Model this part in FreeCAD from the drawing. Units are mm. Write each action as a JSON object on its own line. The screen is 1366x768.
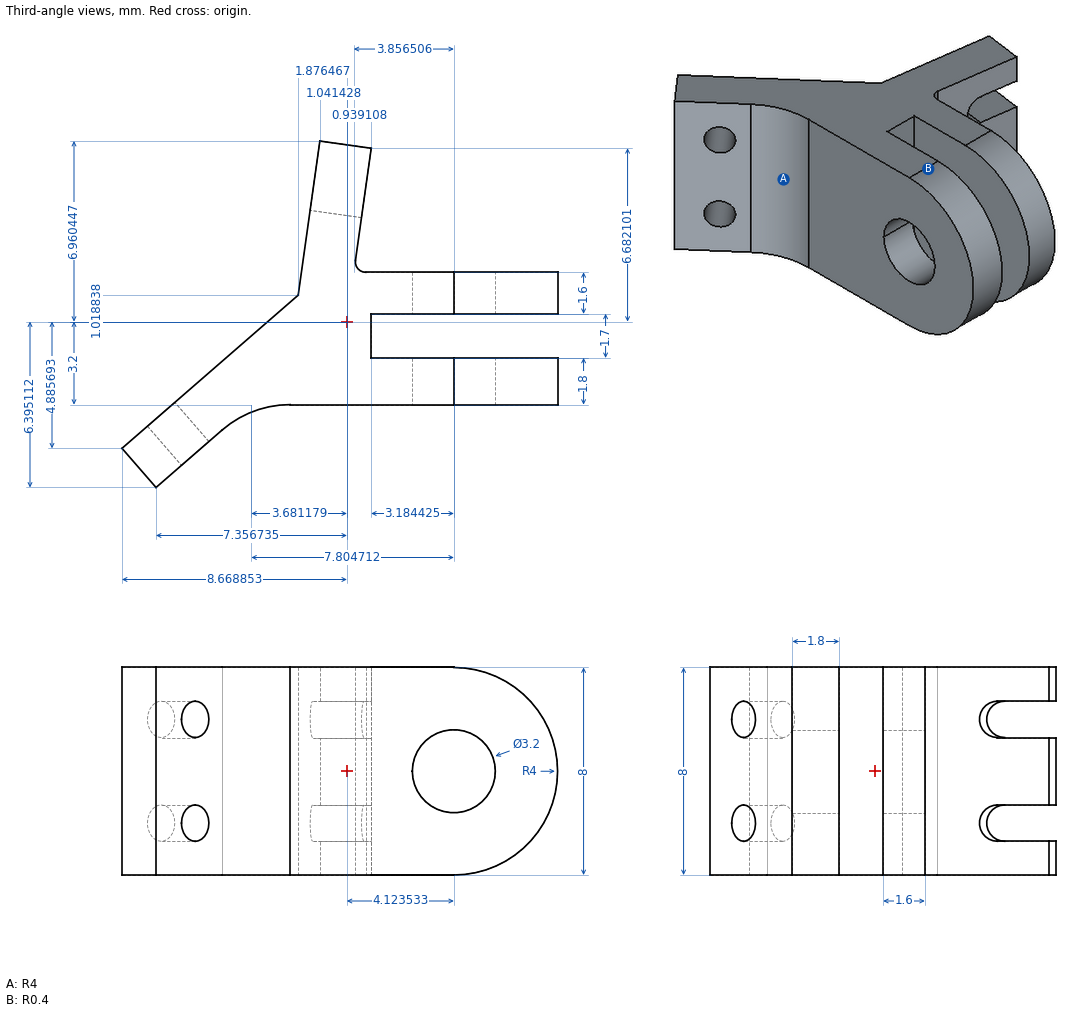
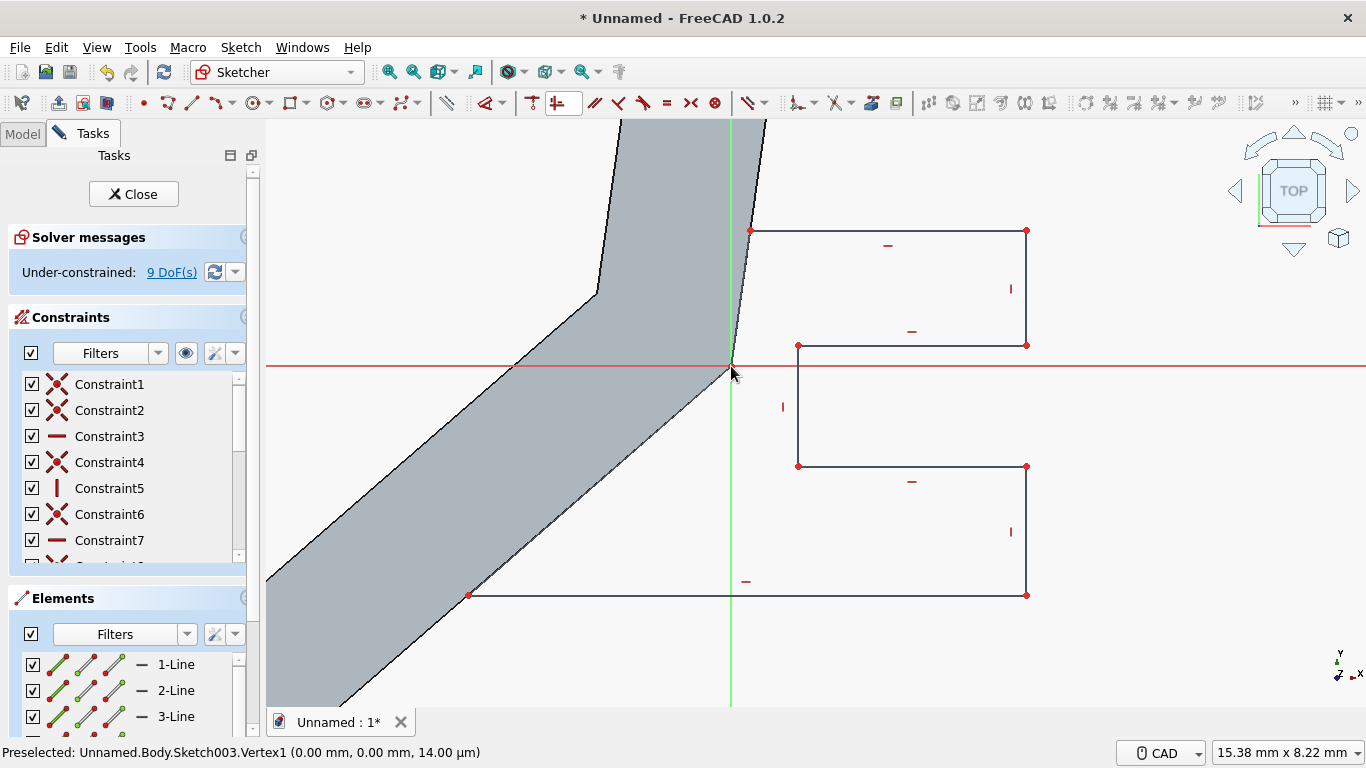
{"action": "left_click", "coordinate": [486, 104]}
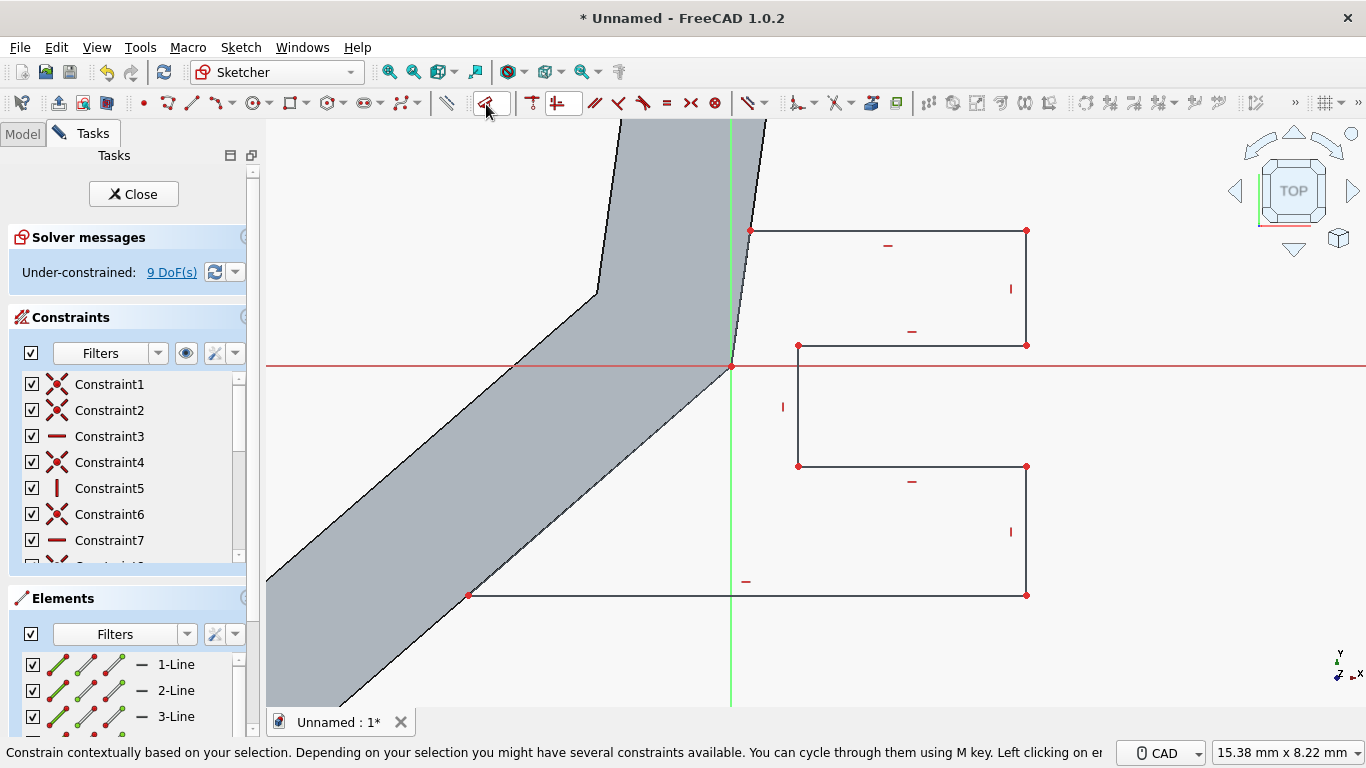
{"action": "left_click", "coordinate": [1026, 557]}
{"action": "left_click", "coordinate": [1060, 532]}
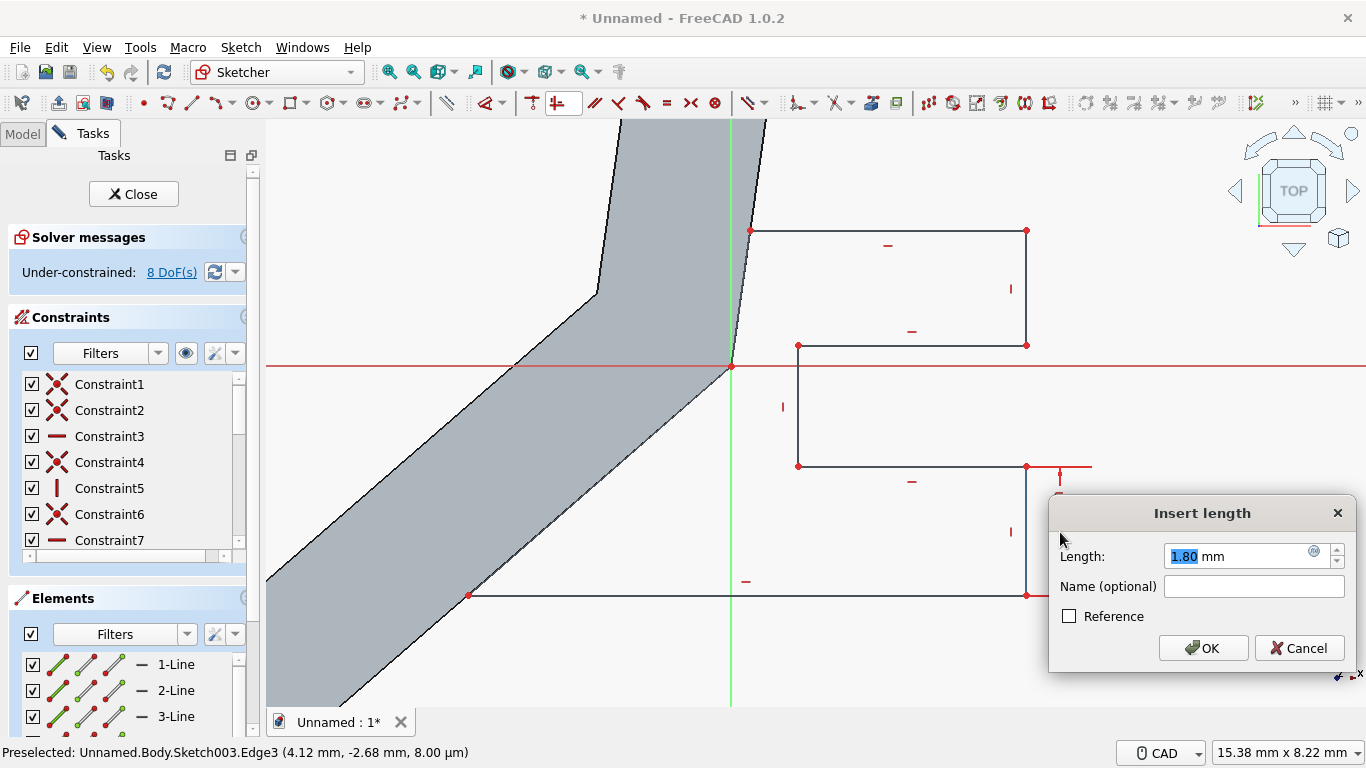
{"action": "type", "text": "1.8"}
{"action": "key", "text": "Return"}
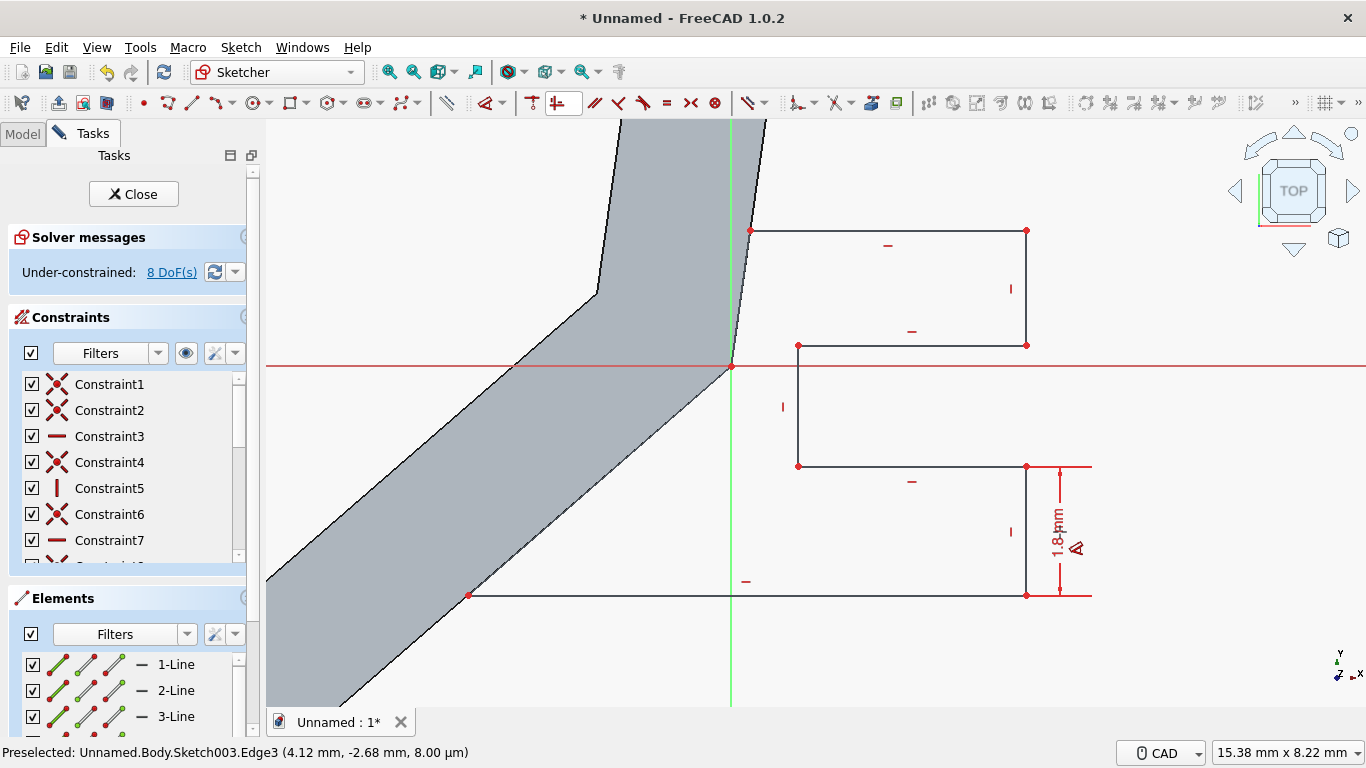
{"action": "left_click", "coordinate": [798, 431]}
{"action": "left_click", "coordinate": [832, 407]}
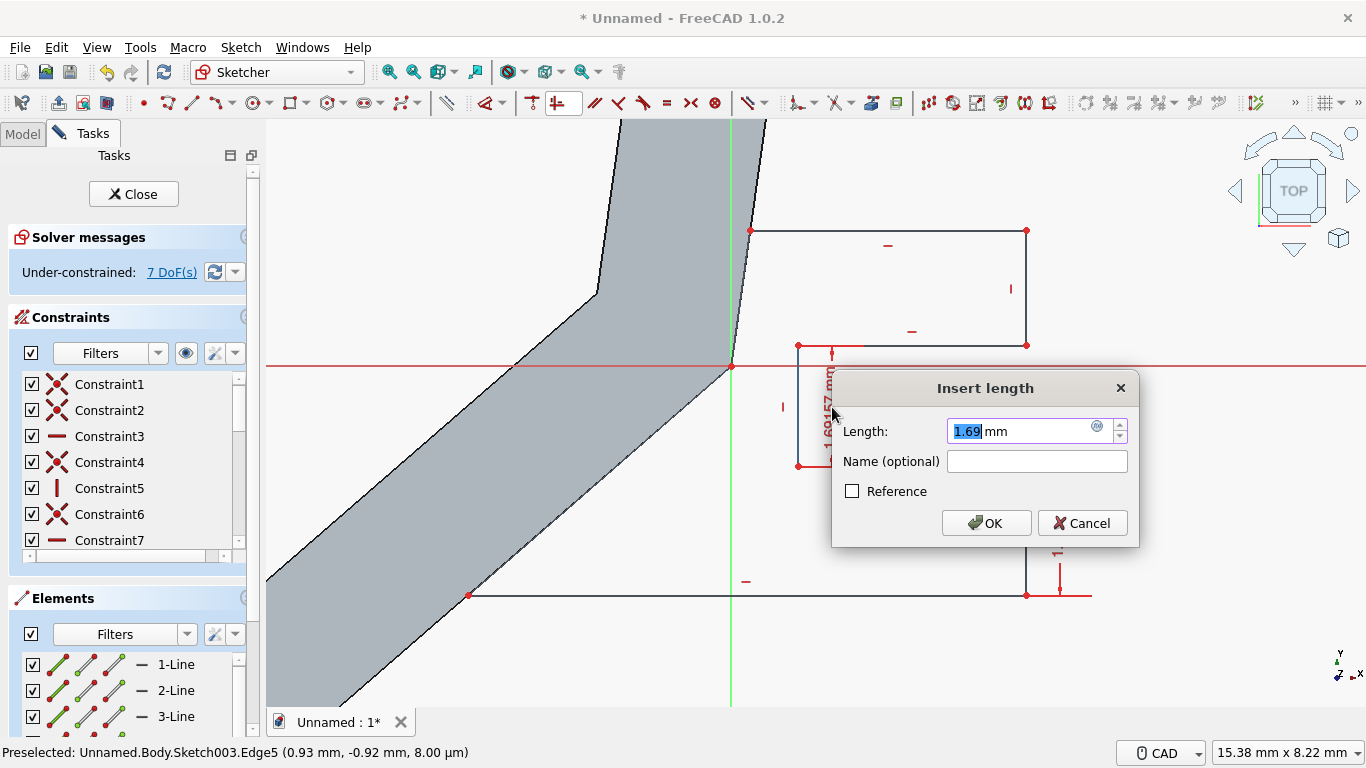
{"action": "type", "text": "1.7"}
{"action": "key", "text": "Return"}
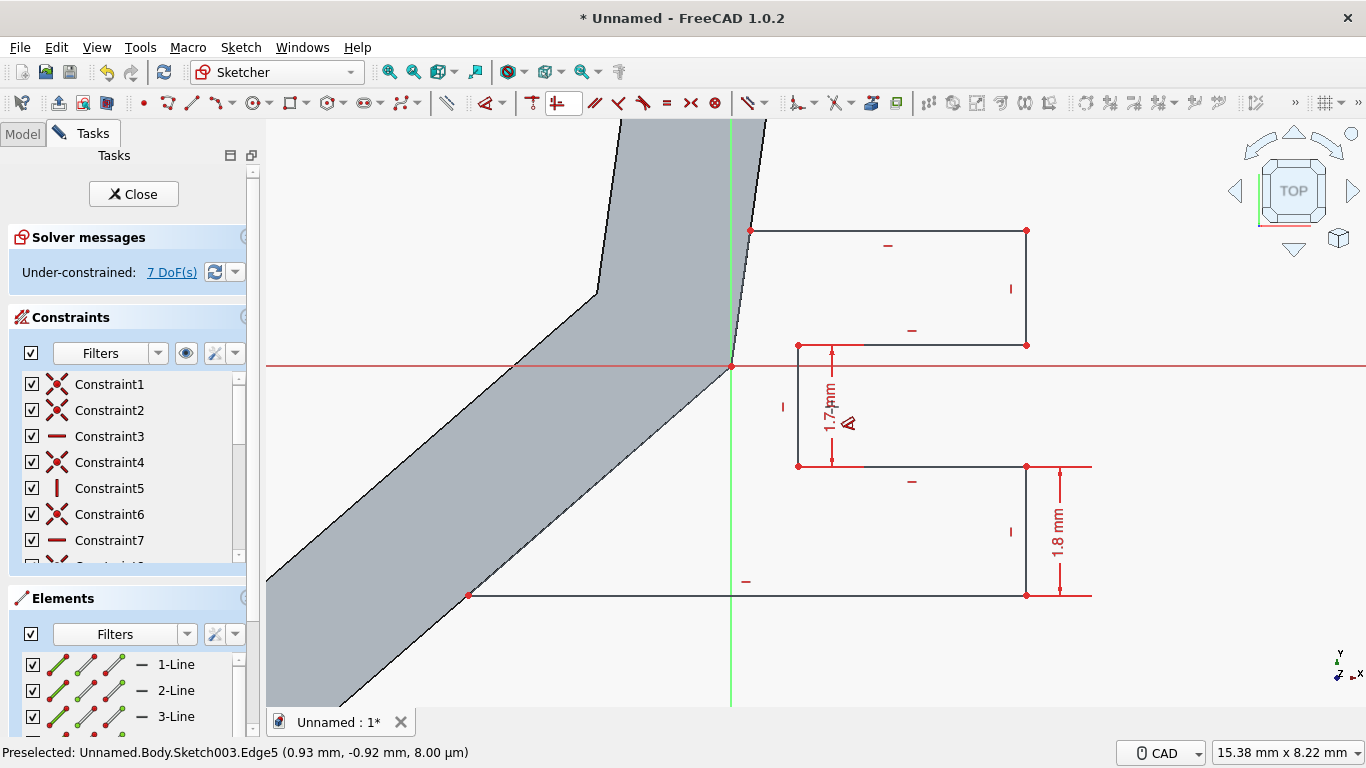
{"action": "left_click", "coordinate": [1026, 311]}
{"action": "left_click", "coordinate": [1060, 288]}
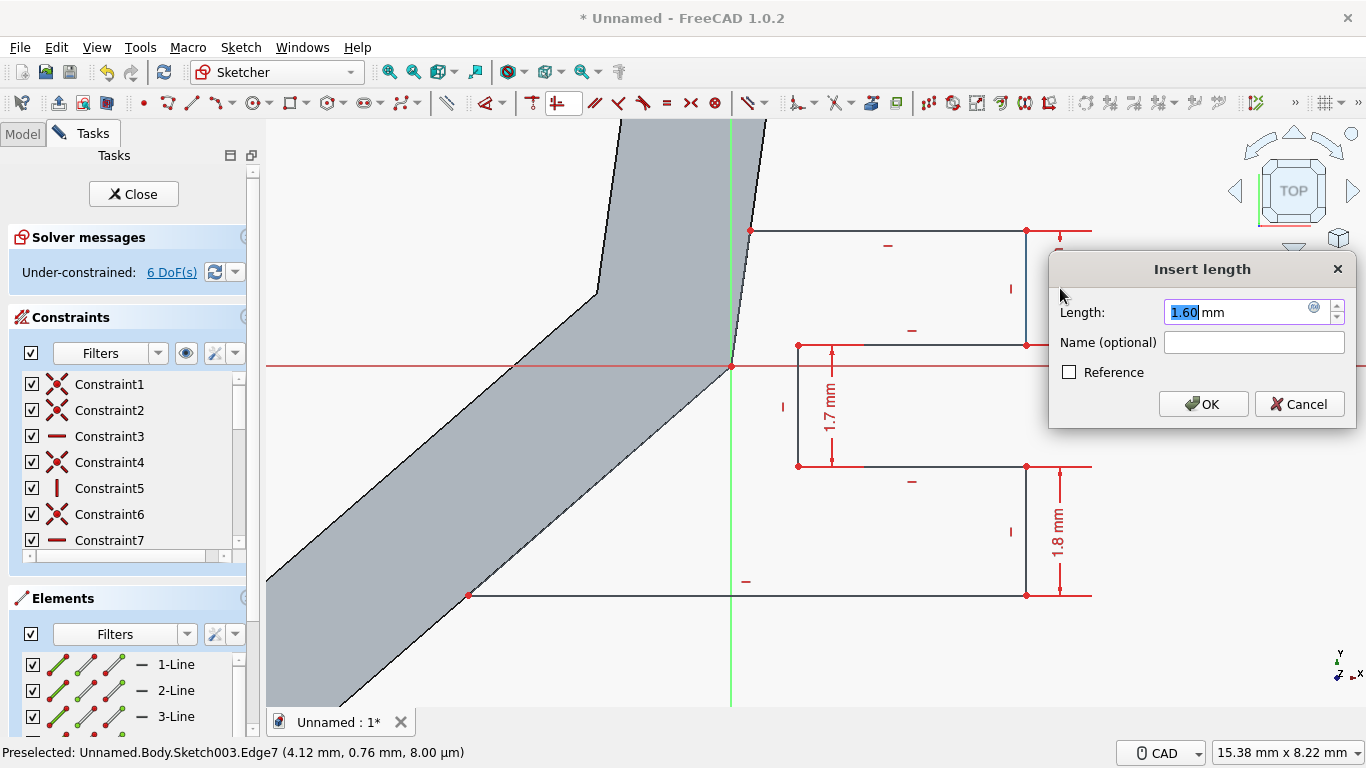
{"action": "type", "text": "1.6"}
{"action": "key", "text": "Return"}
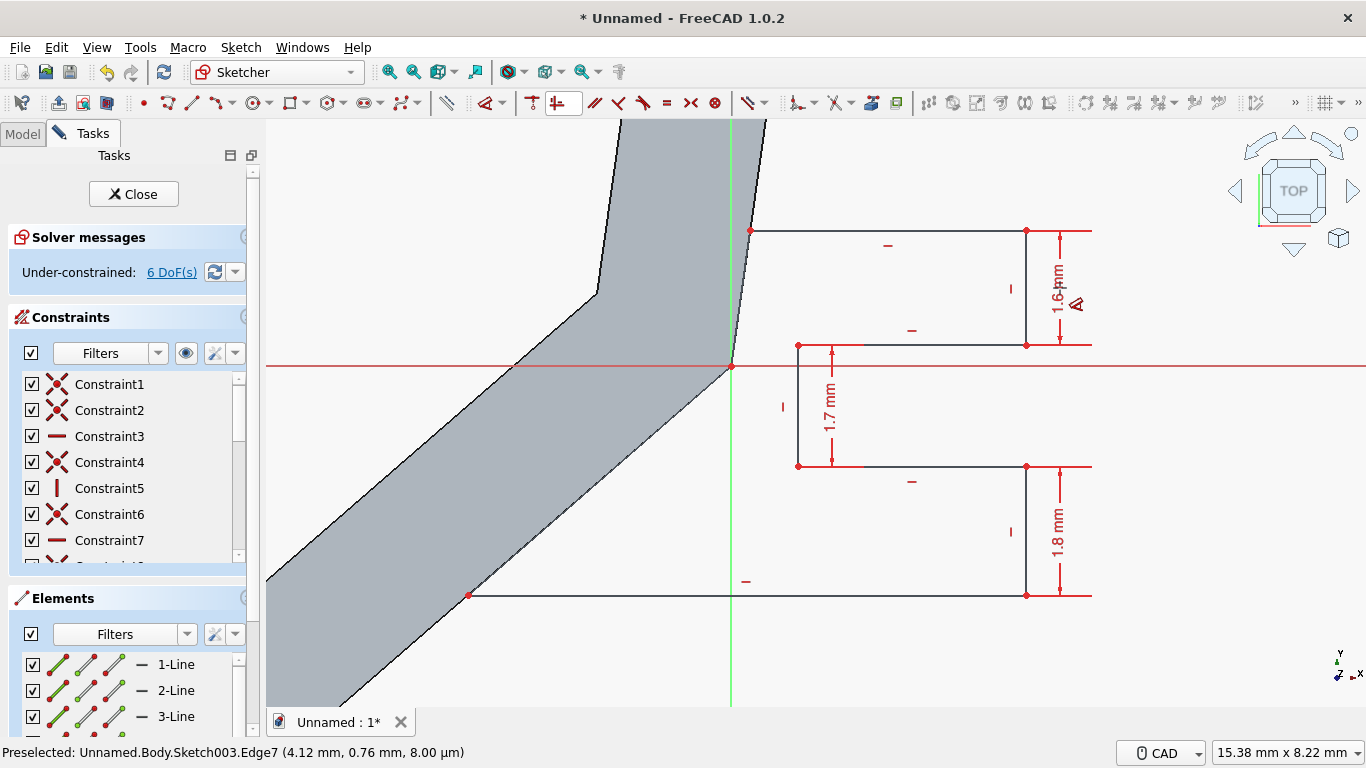
{"action": "left_click", "coordinate": [468, 596]}
{"action": "left_click", "coordinate": [434, 481]}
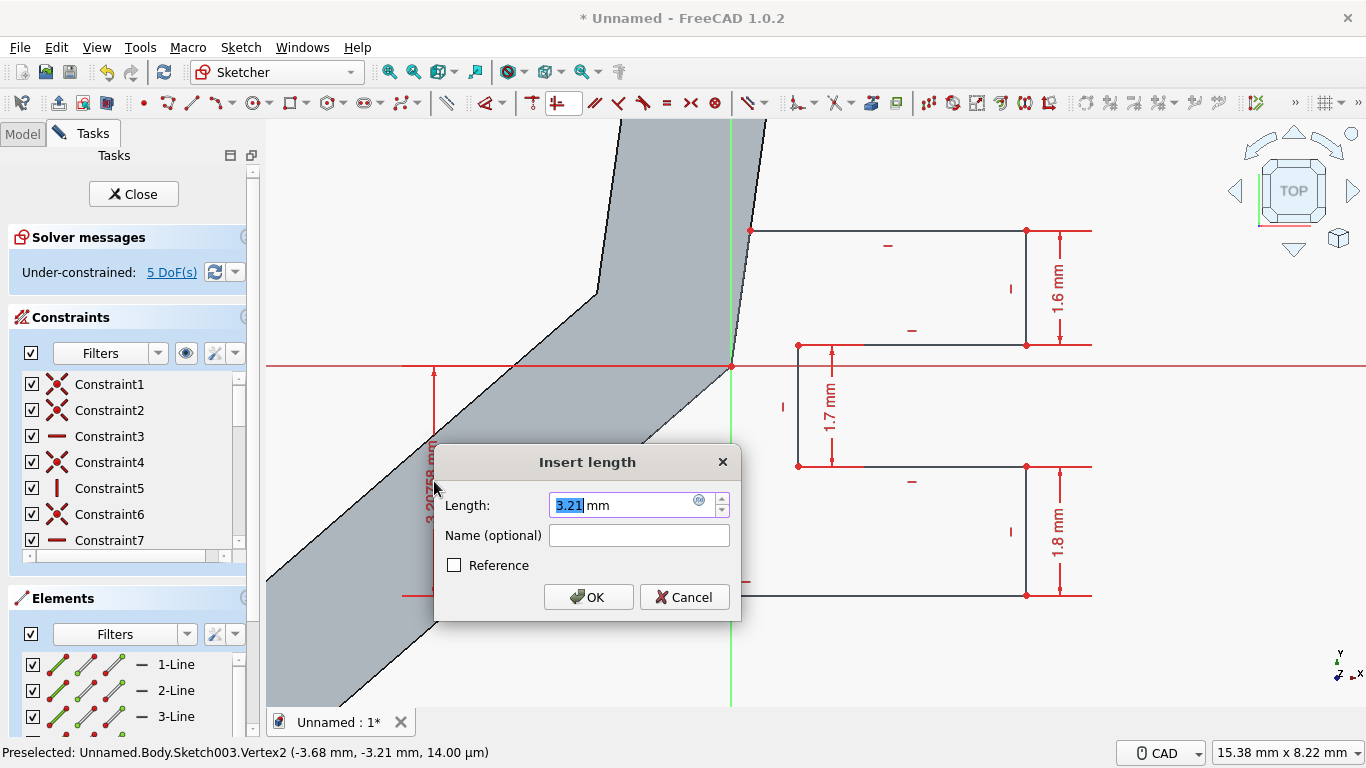
{"action": "type", "text": "3.2"}
{"action": "key", "text": "Return"}